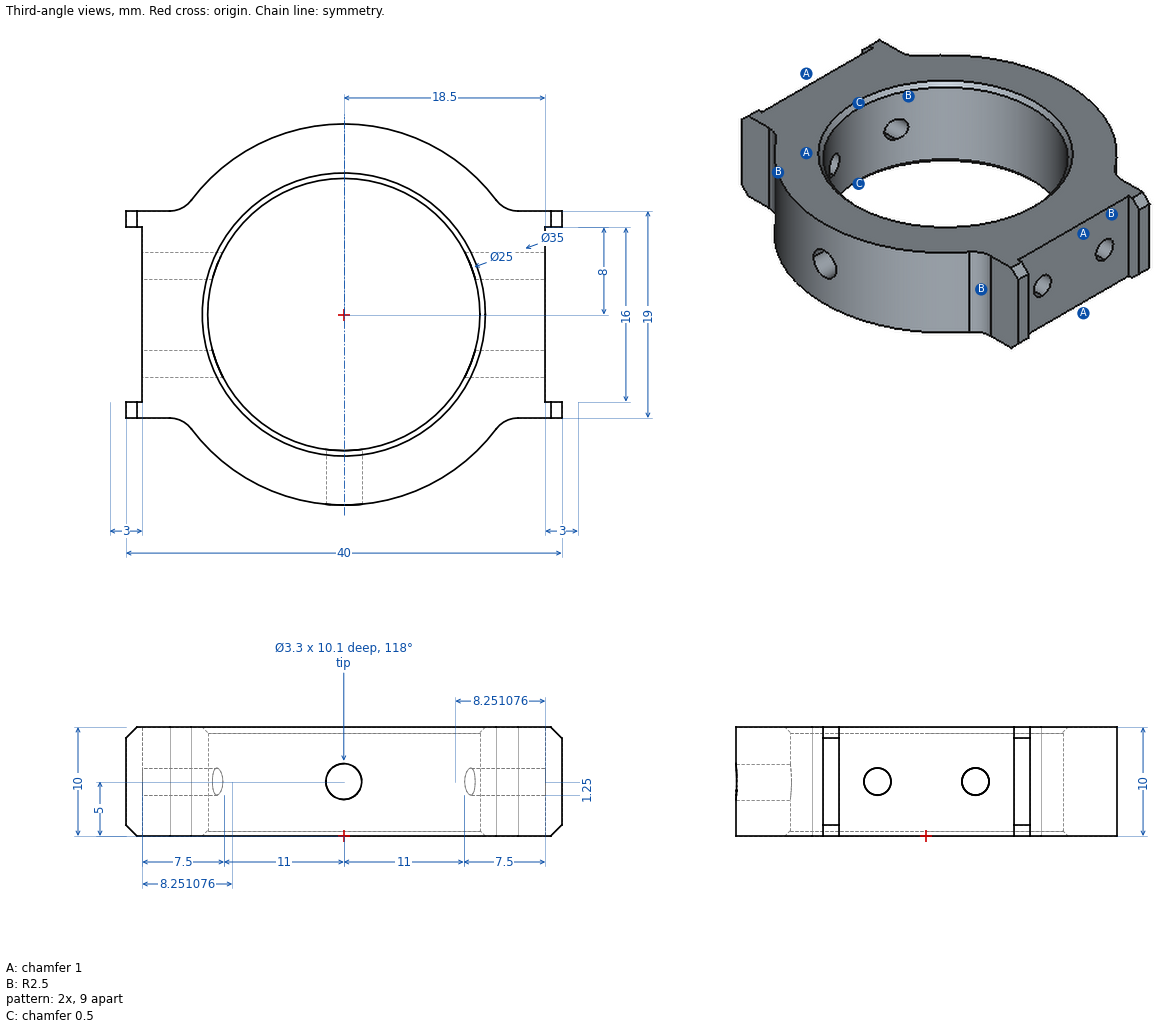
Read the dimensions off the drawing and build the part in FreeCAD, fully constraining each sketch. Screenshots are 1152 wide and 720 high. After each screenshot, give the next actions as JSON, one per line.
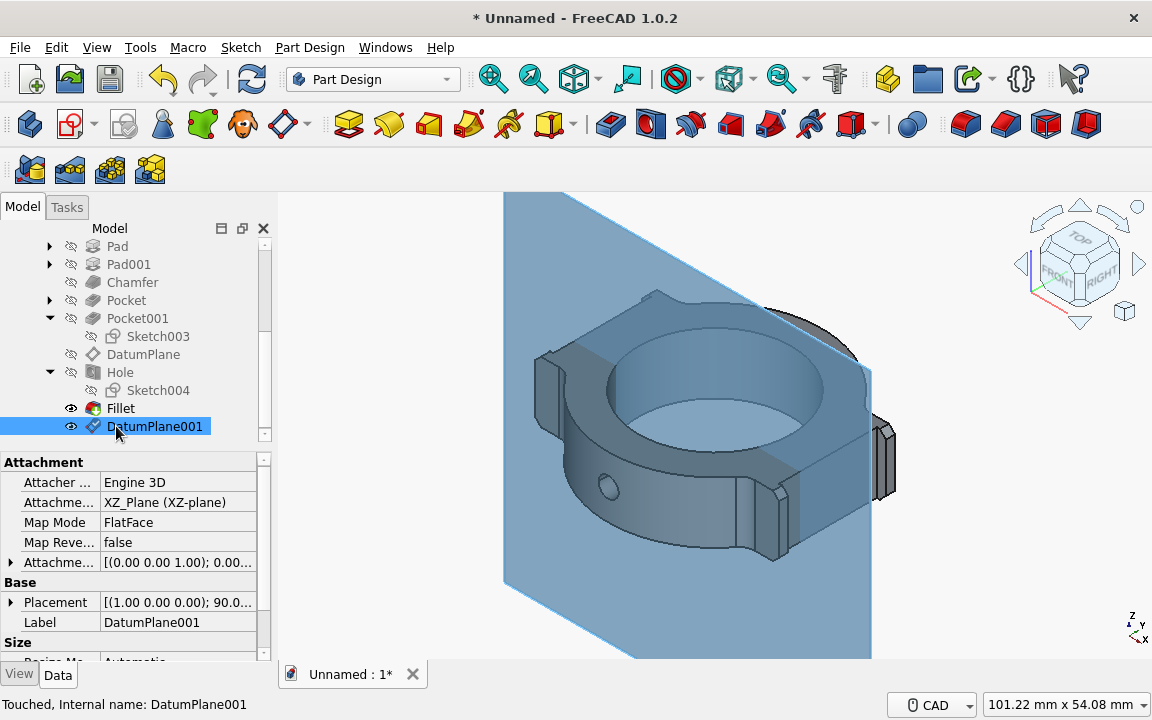
{"action": "left_click", "coordinate": [70, 124]}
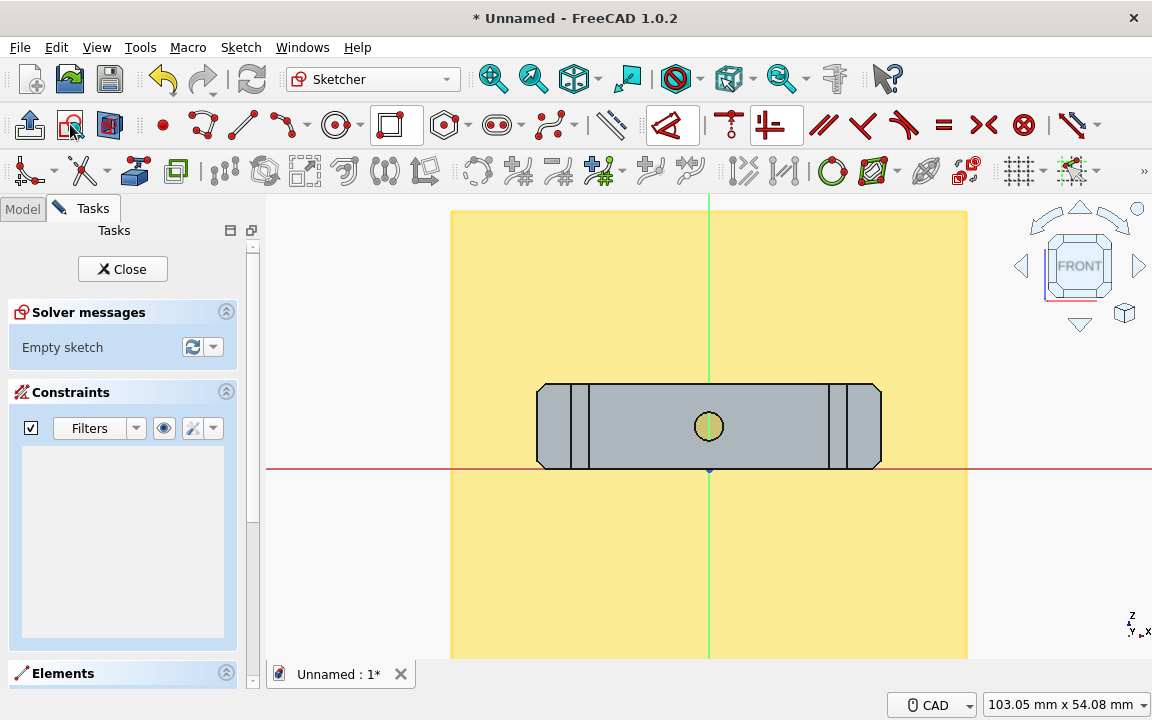
{"action": "left_click", "coordinate": [110, 126]}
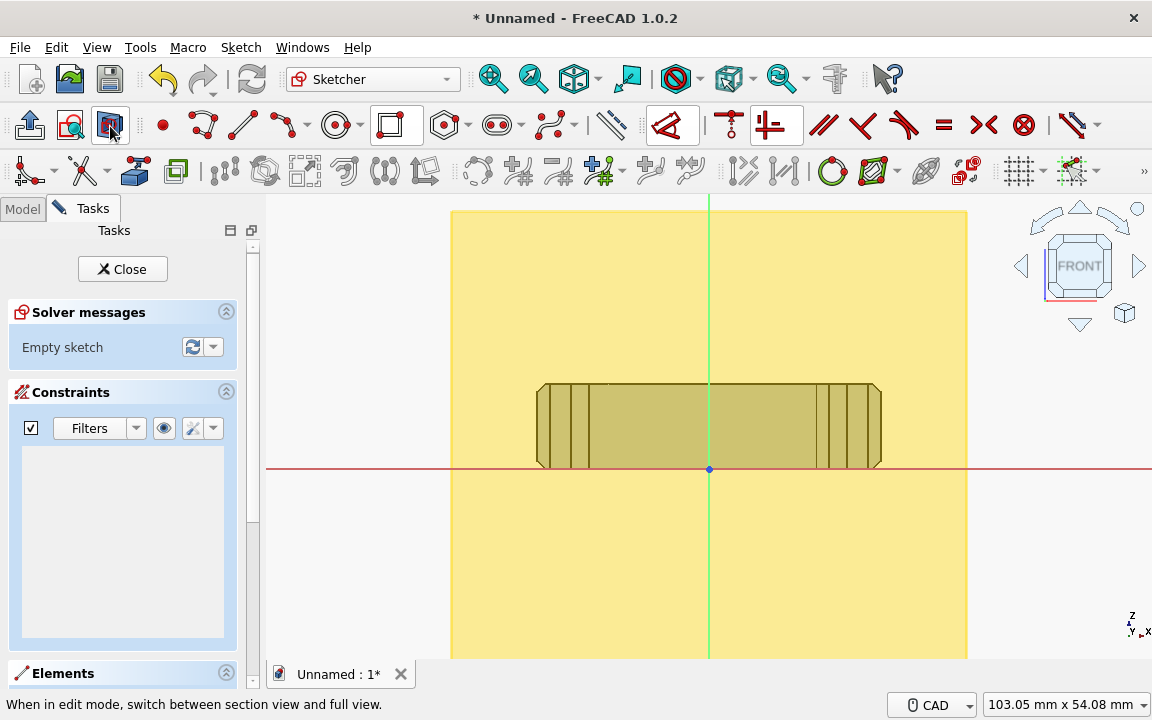
{"action": "scroll", "coordinate": [852, 457], "scroll_direction": "up", "scroll_amount": 6}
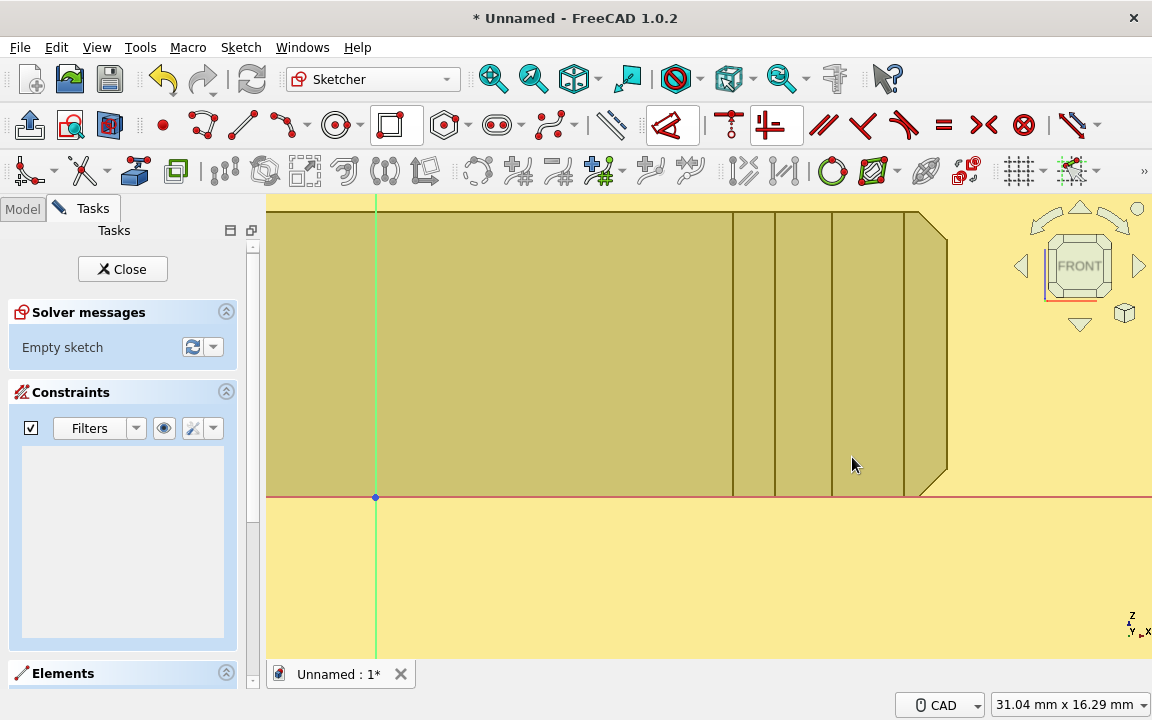
{"action": "left_click", "coordinate": [204, 126]}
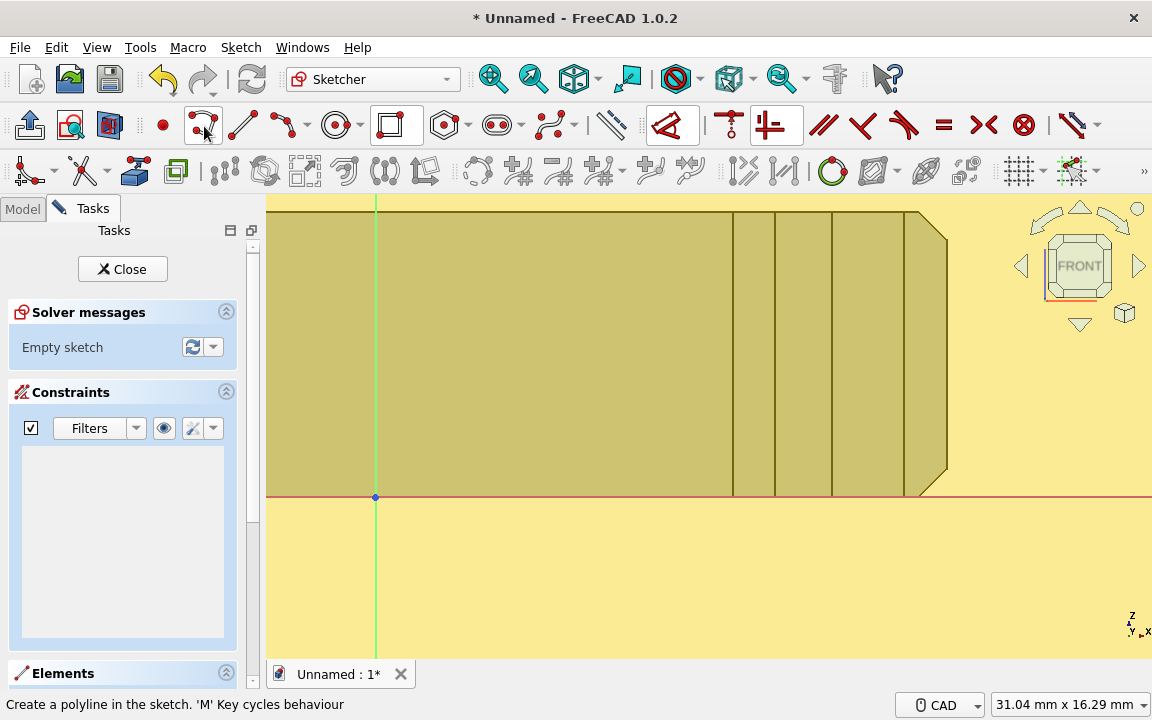
{"action": "left_click", "coordinate": [668, 354]}
{"action": "left_click", "coordinate": [904, 354]}
{"action": "left_click", "coordinate": [904, 390]}
{"action": "left_click", "coordinate": [690, 390]}
{"action": "left_click", "coordinate": [668, 355]}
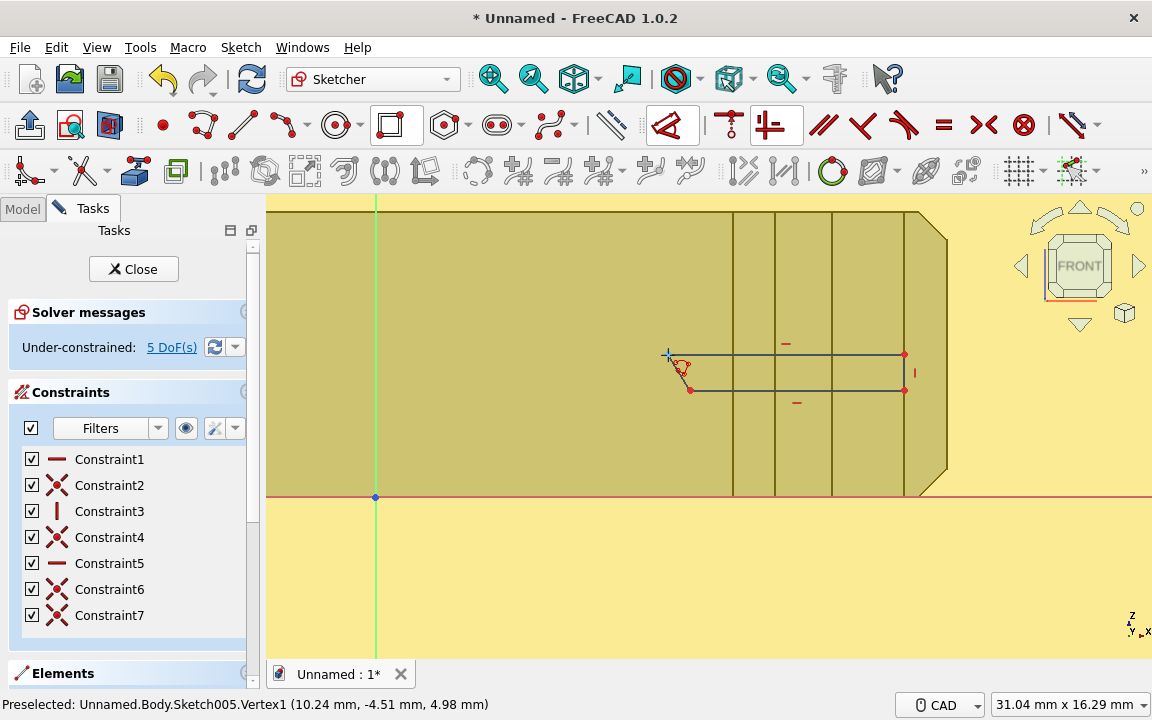
{"action": "left_click", "coordinate": [244, 126]}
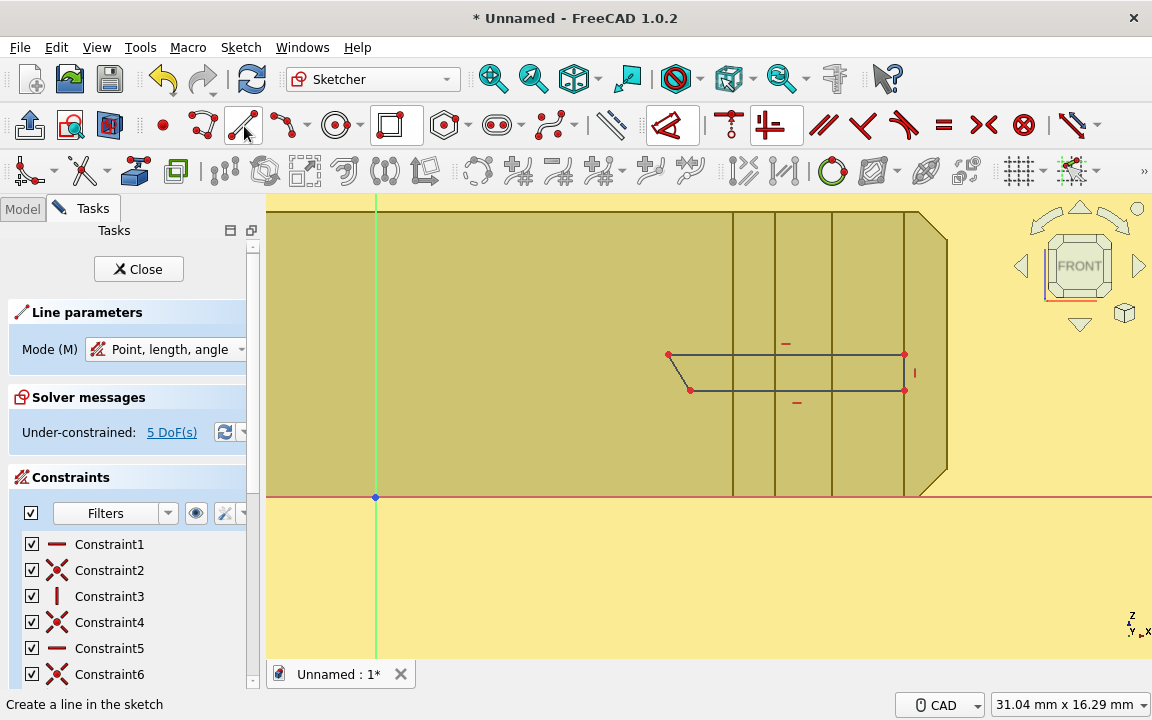
{"action": "left_click", "coordinate": [645, 354]}
{"action": "left_click", "coordinate": [574, 354]}
{"action": "key", "text": "Escape"}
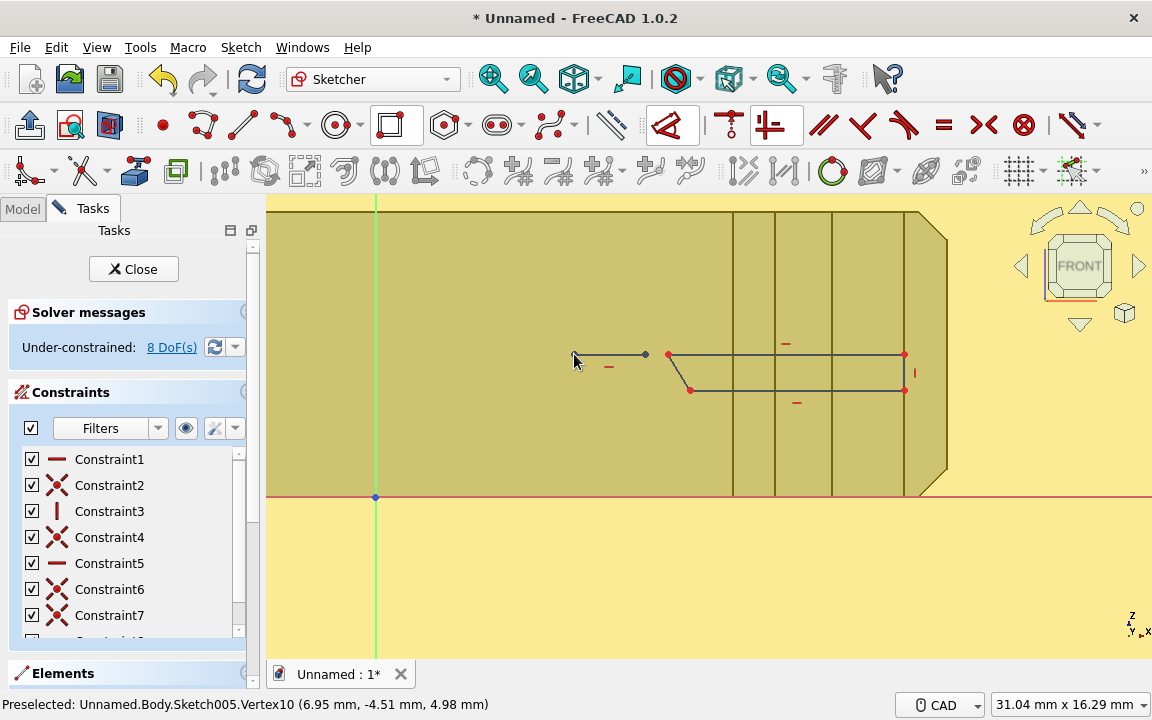
{"action": "left_click", "coordinate": [624, 355]}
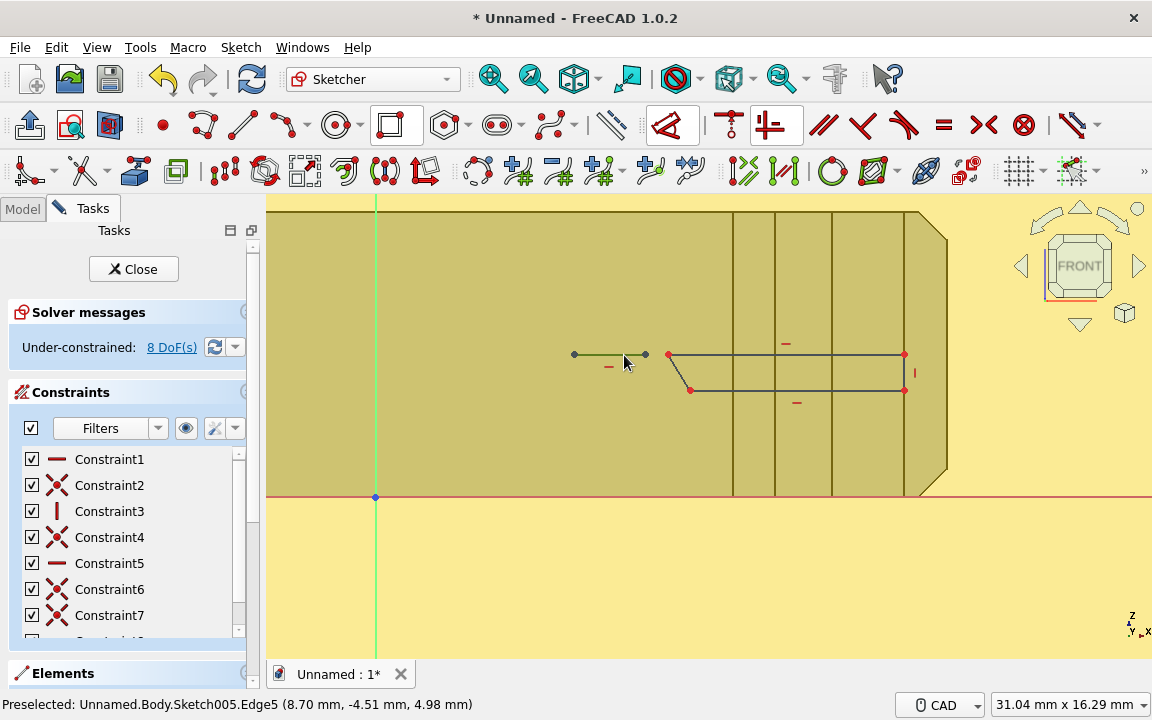
{"action": "left_click", "coordinate": [612, 126]}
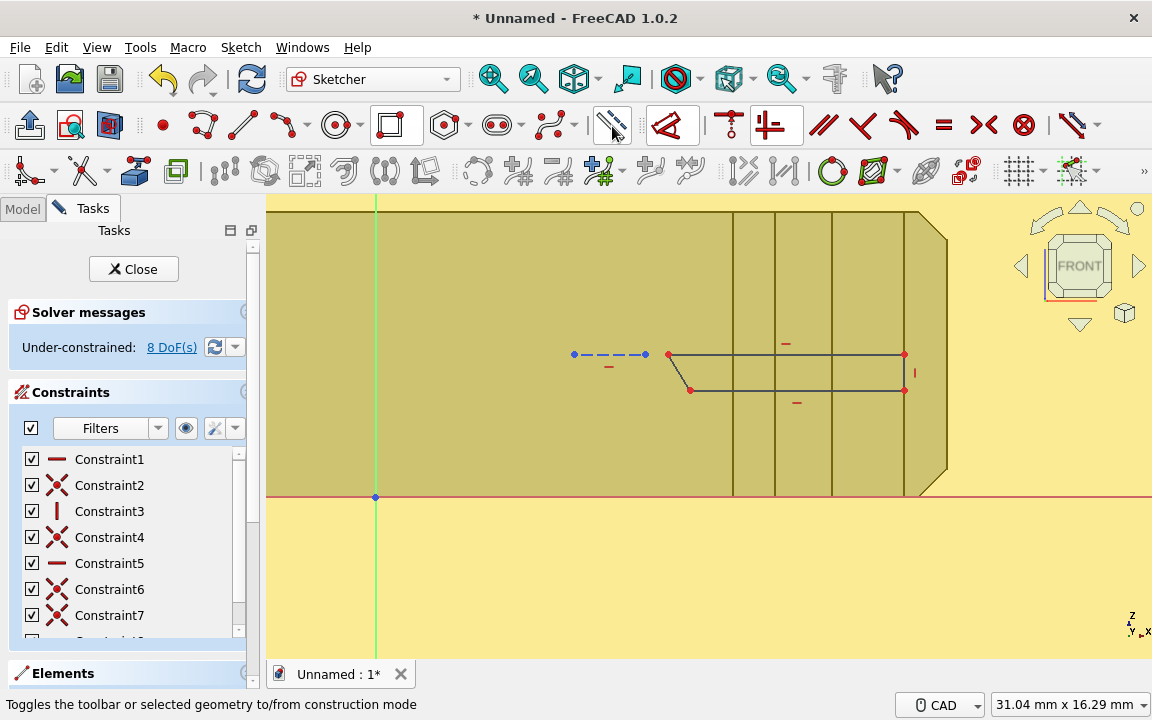
{"action": "left_click", "coordinate": [668, 355]}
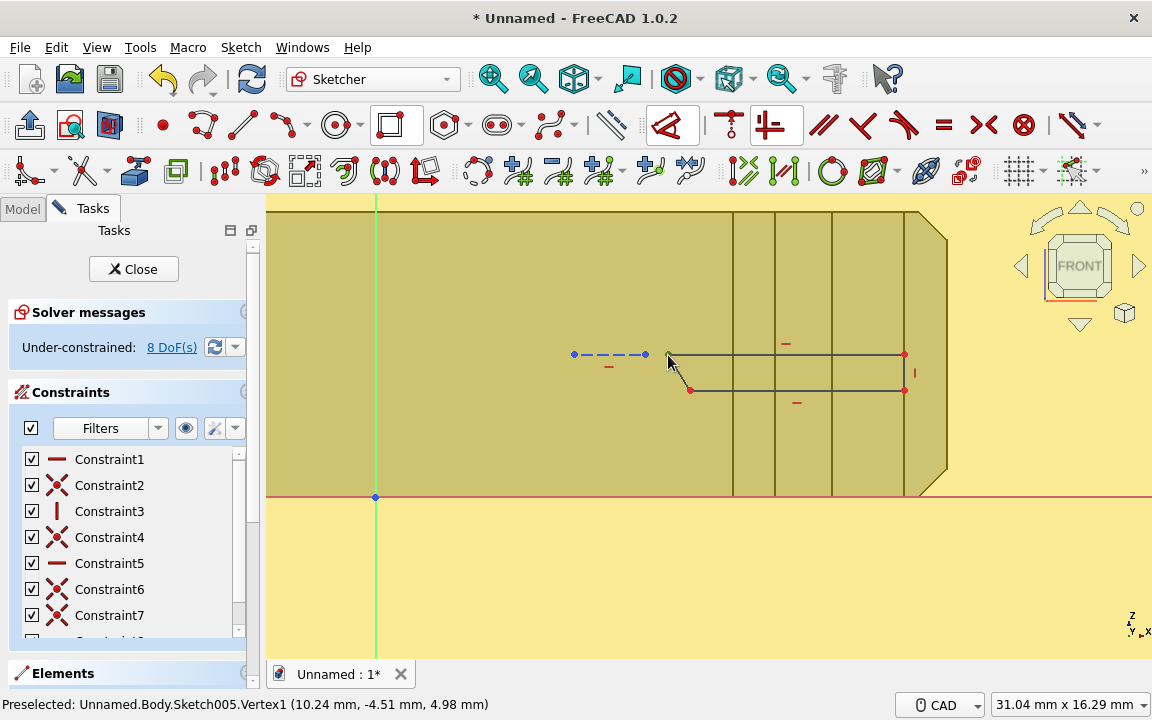
{"action": "left_click", "coordinate": [694, 126]}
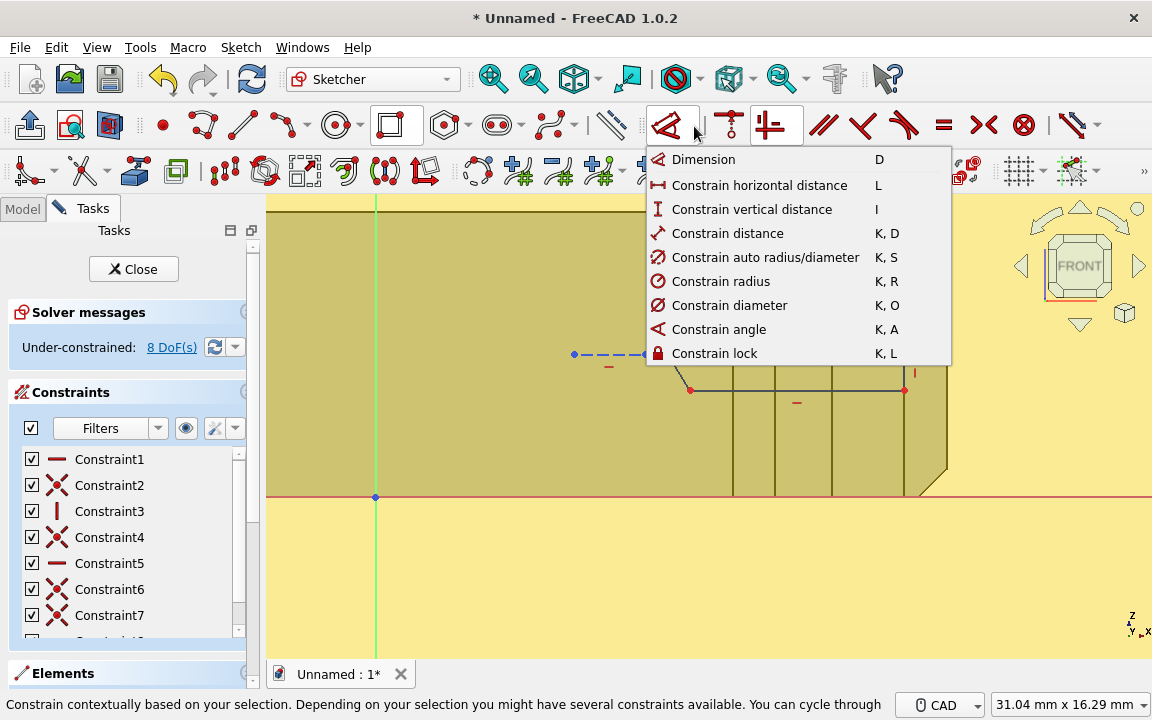
{"action": "left_click", "coordinate": [799, 209]}